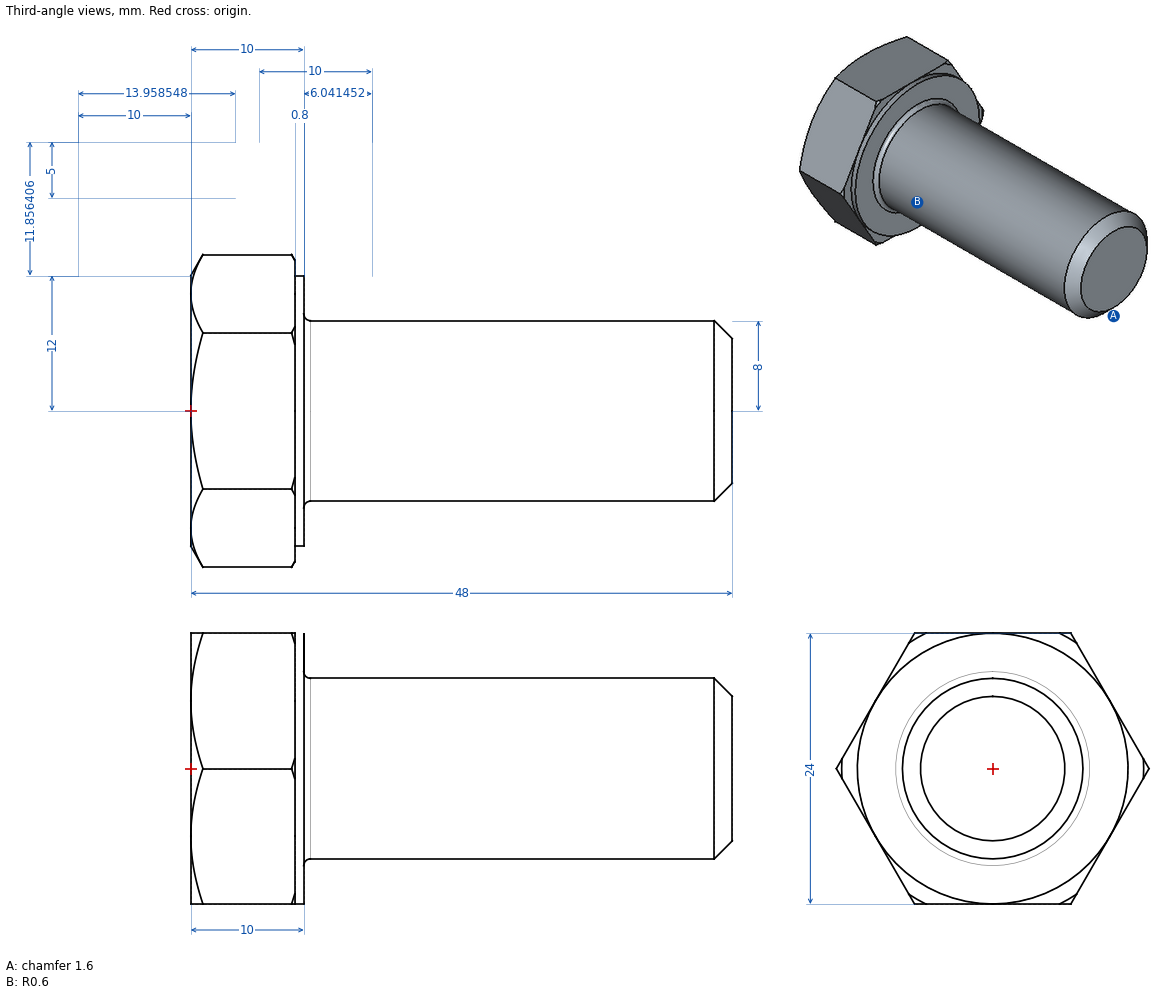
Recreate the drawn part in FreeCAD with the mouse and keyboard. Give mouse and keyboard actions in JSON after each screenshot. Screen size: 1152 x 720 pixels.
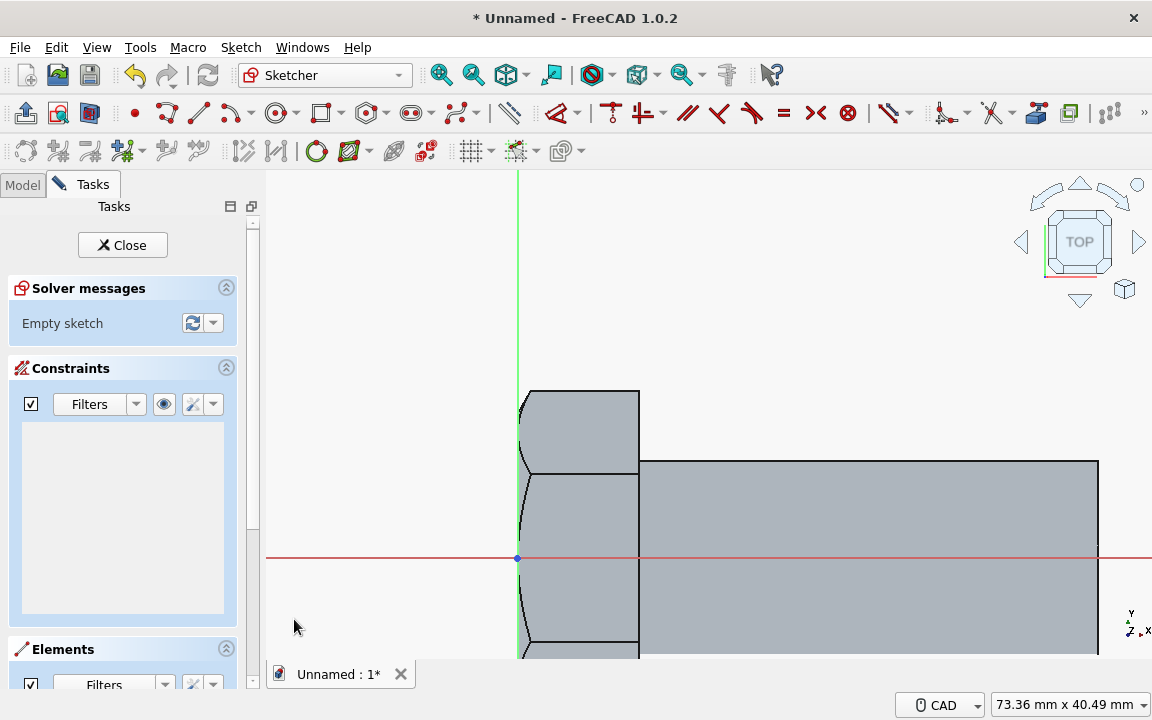
{"action": "left_click", "coordinate": [168, 114]}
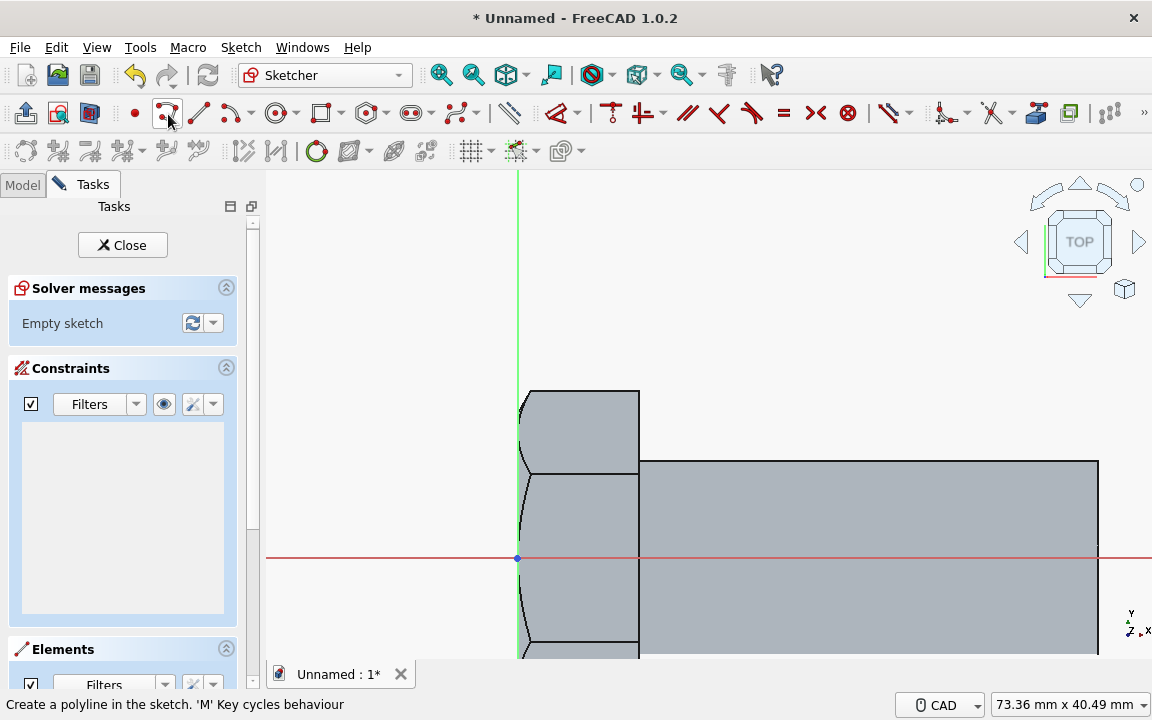
{"action": "left_click", "coordinate": [639, 413]}
{"action": "left_click", "coordinate": [712, 413]}
{"action": "left_click", "coordinate": [712, 270]}
{"action": "left_click", "coordinate": [591, 270]}
{"action": "left_click", "coordinate": [591, 330]}
{"action": "left_click", "coordinate": [639, 414]}
{"action": "key", "text": "Escape"}
{"action": "key", "text": "Escape"}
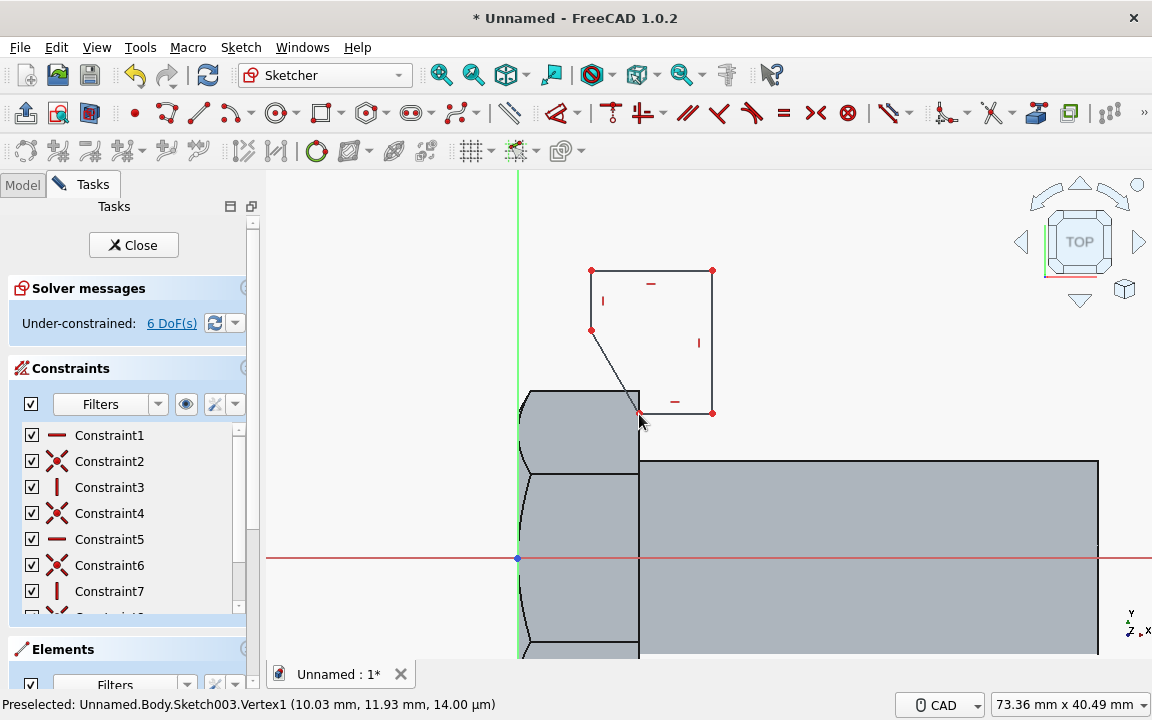
{"action": "left_click", "coordinate": [556, 114]}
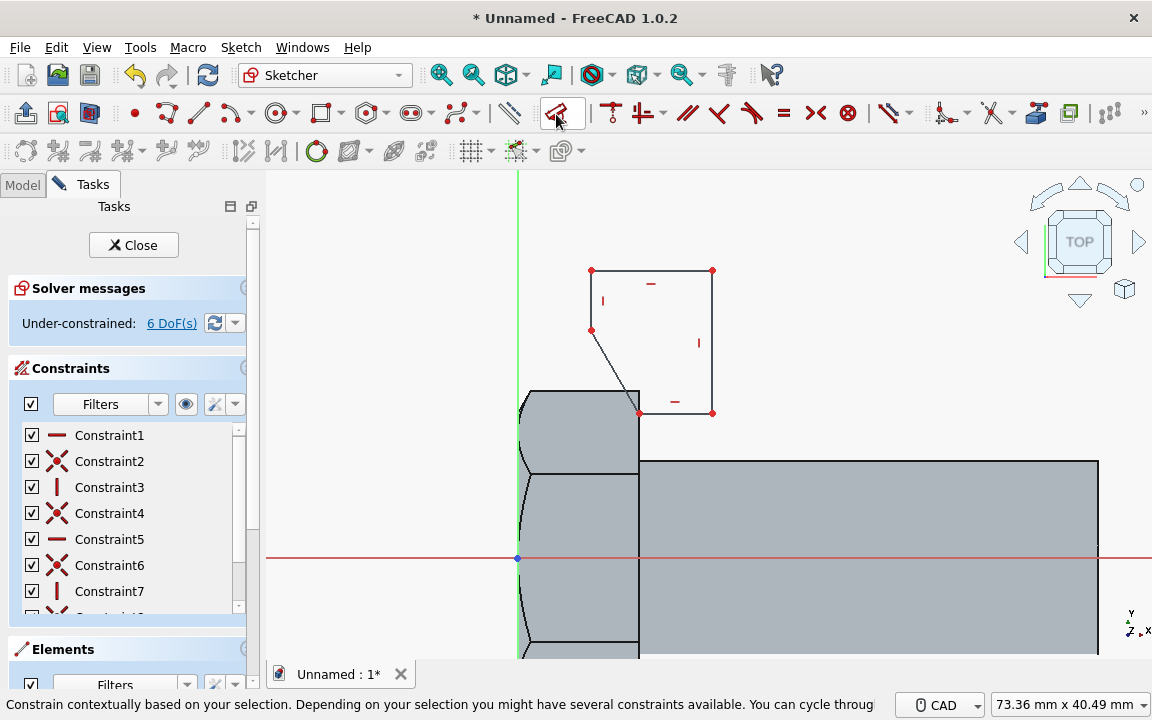
{"action": "left_click", "coordinate": [591, 289]}
{"action": "left_click", "coordinate": [557, 301]}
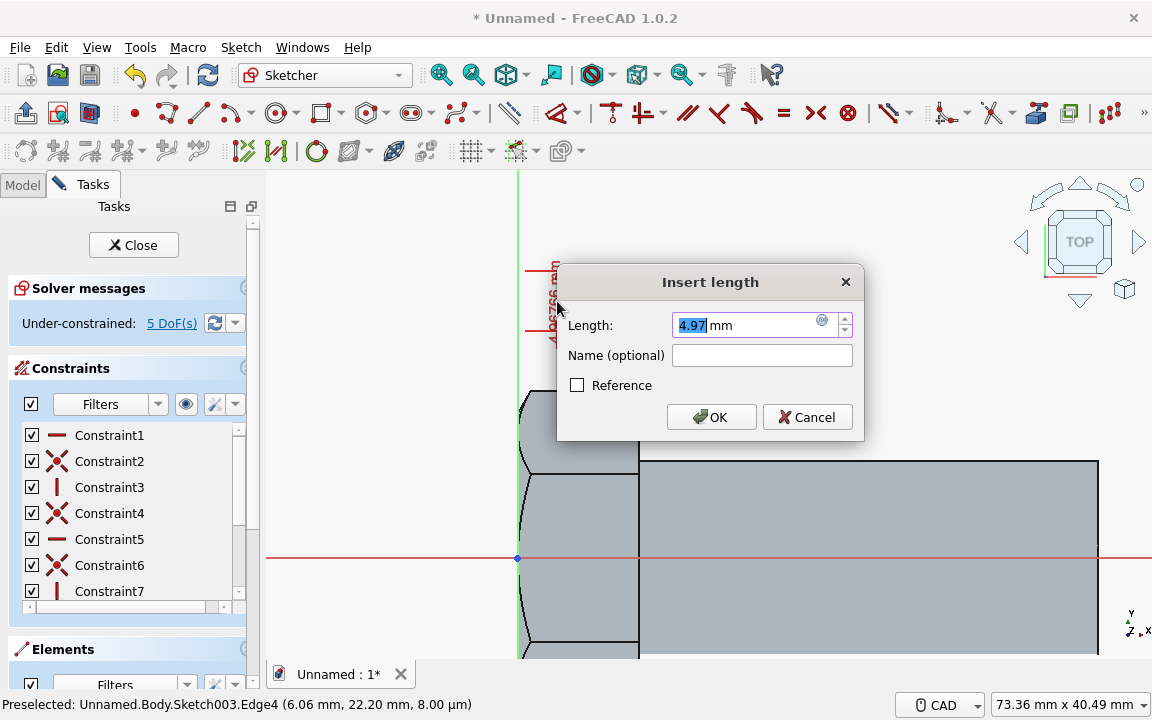
{"action": "type", "text": "5"}
{"action": "key", "text": "Return"}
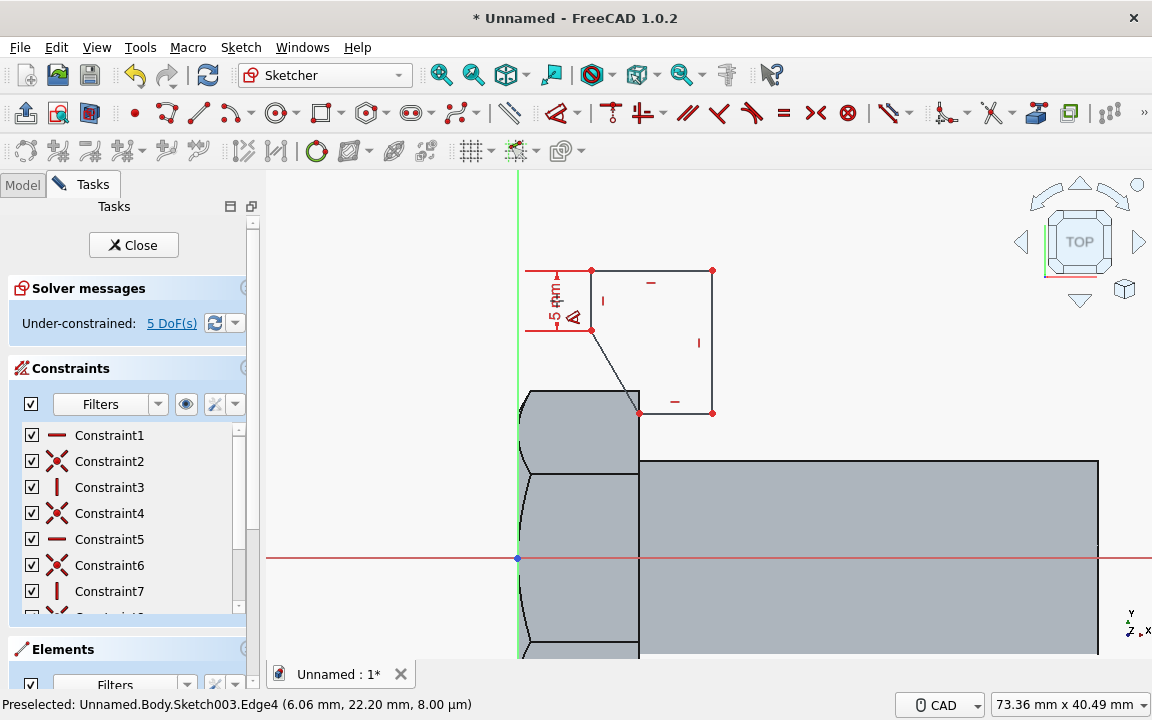
{"action": "left_click", "coordinate": [676, 271]}
{"action": "left_click", "coordinate": [652, 237]}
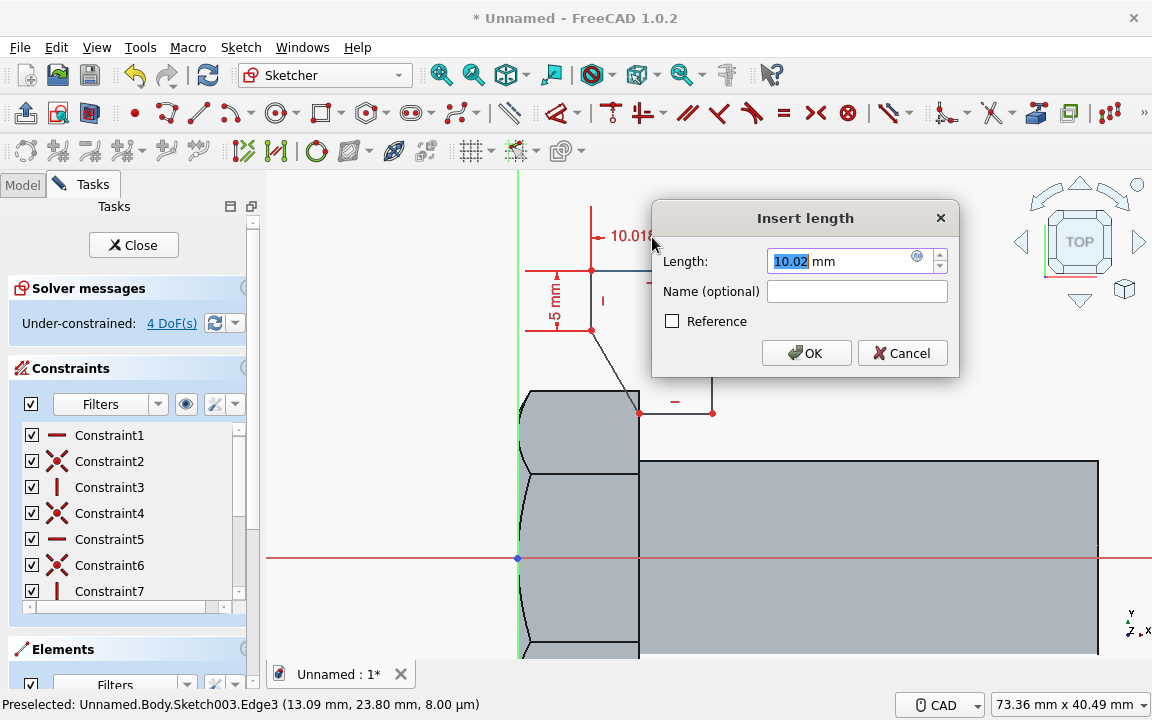
{"action": "type", "text": "10"}
{"action": "key", "text": "Return"}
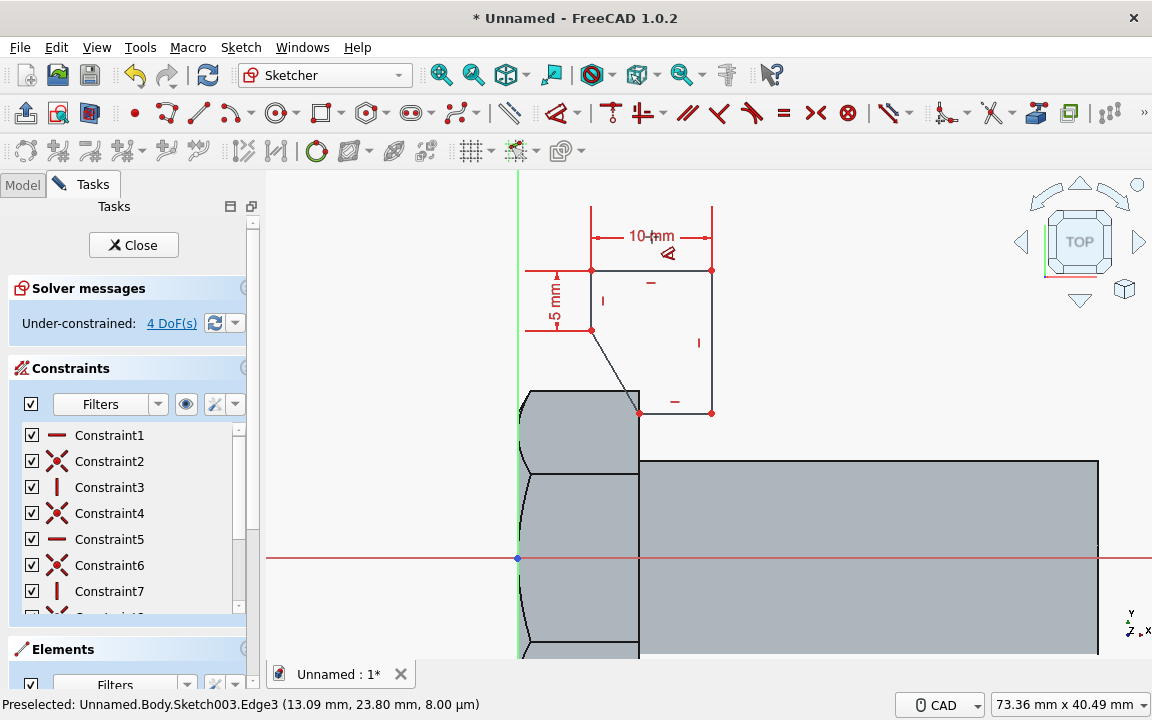
{"action": "left_click", "coordinate": [639, 414]}
{"action": "left_click", "coordinate": [578, 592]}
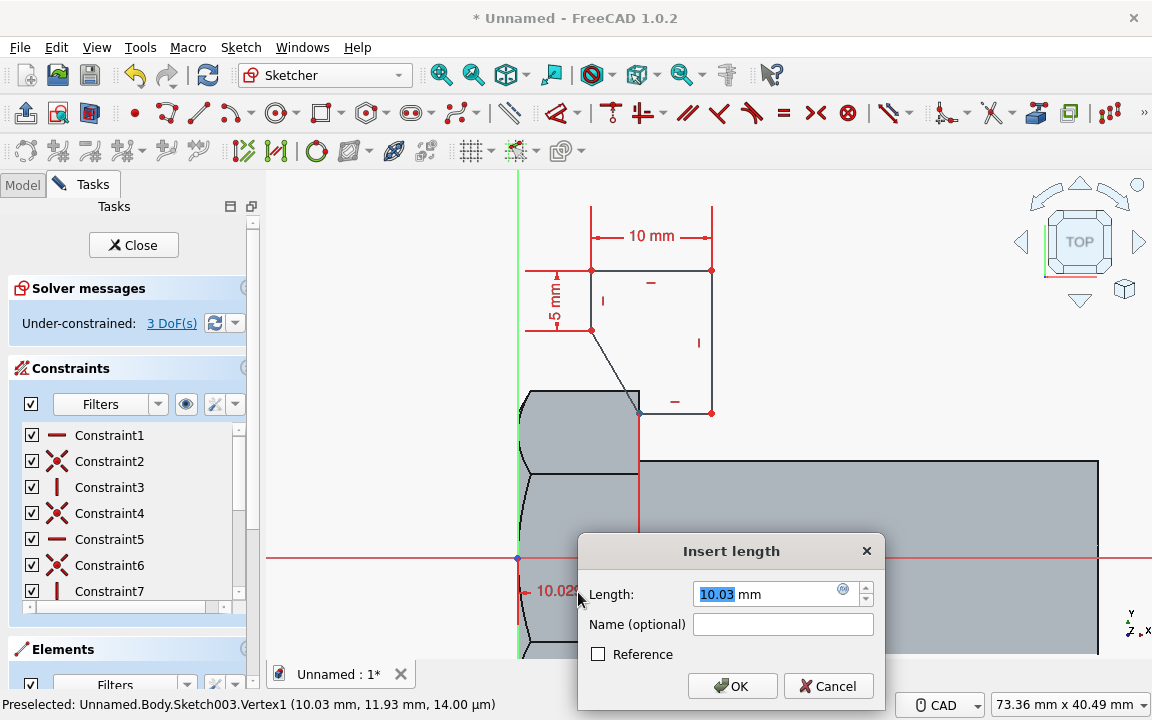
{"action": "type", "text": "10"}
{"action": "key", "text": "Return"}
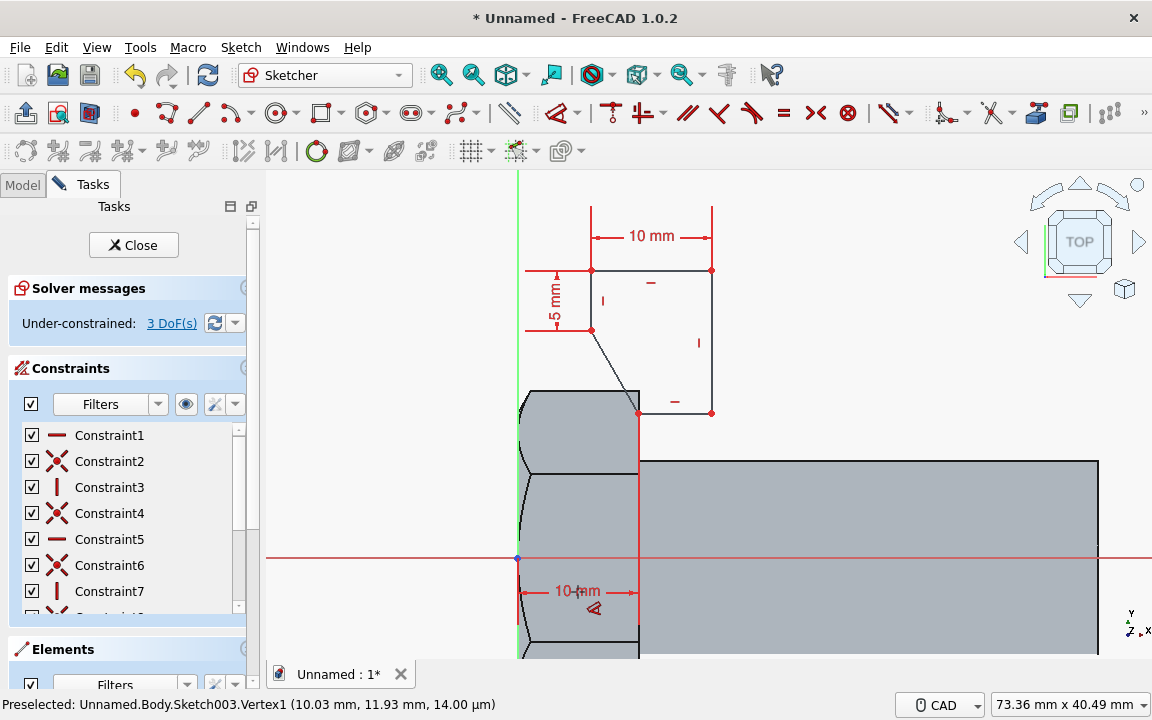
{"action": "left_click", "coordinate": [639, 414]}
{"action": "left_click", "coordinate": [484, 486]}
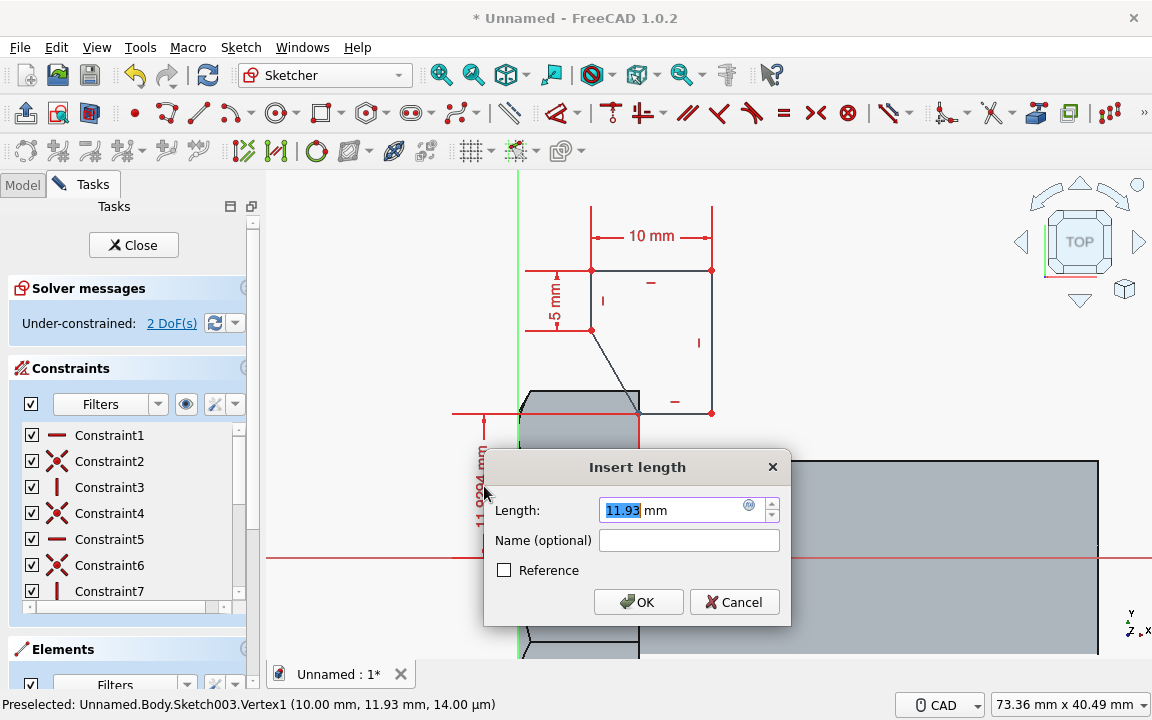
{"action": "type", "text": "12"}
{"action": "key", "text": "Return"}